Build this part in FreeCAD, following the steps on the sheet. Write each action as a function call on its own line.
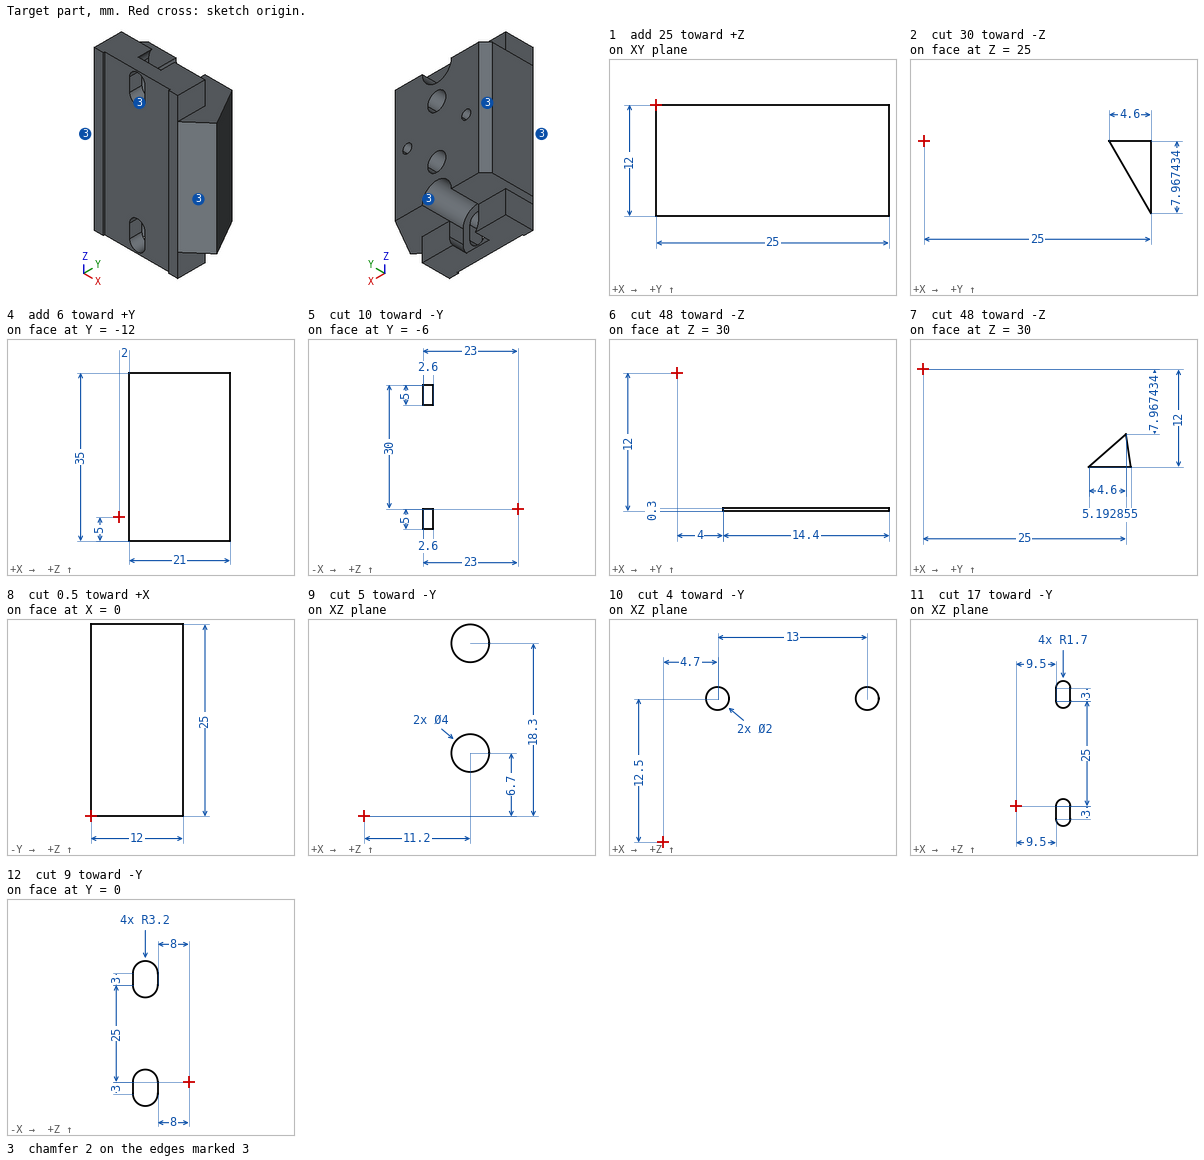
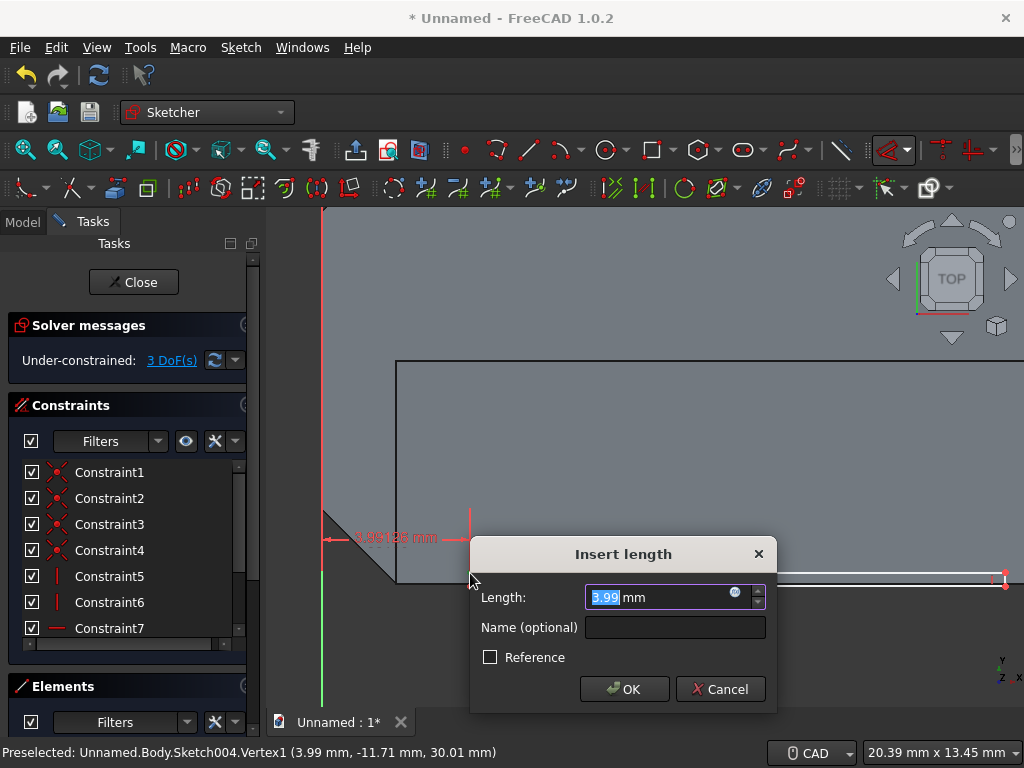
text(4)
key(Return)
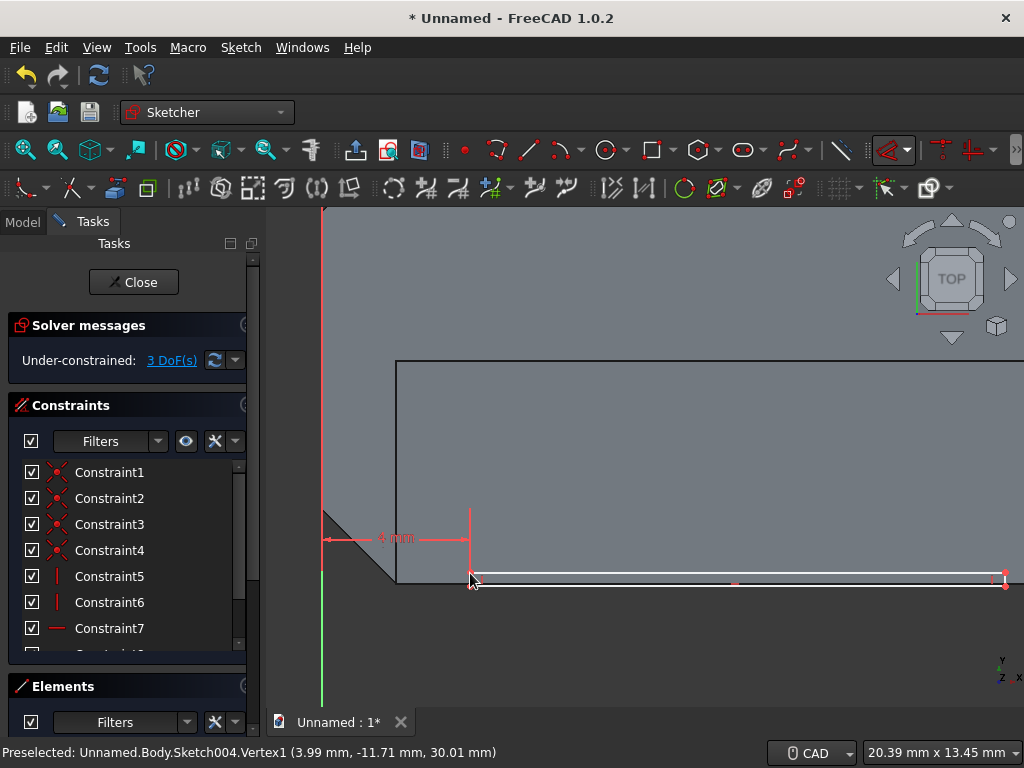
scroll(470, 580, up, 7)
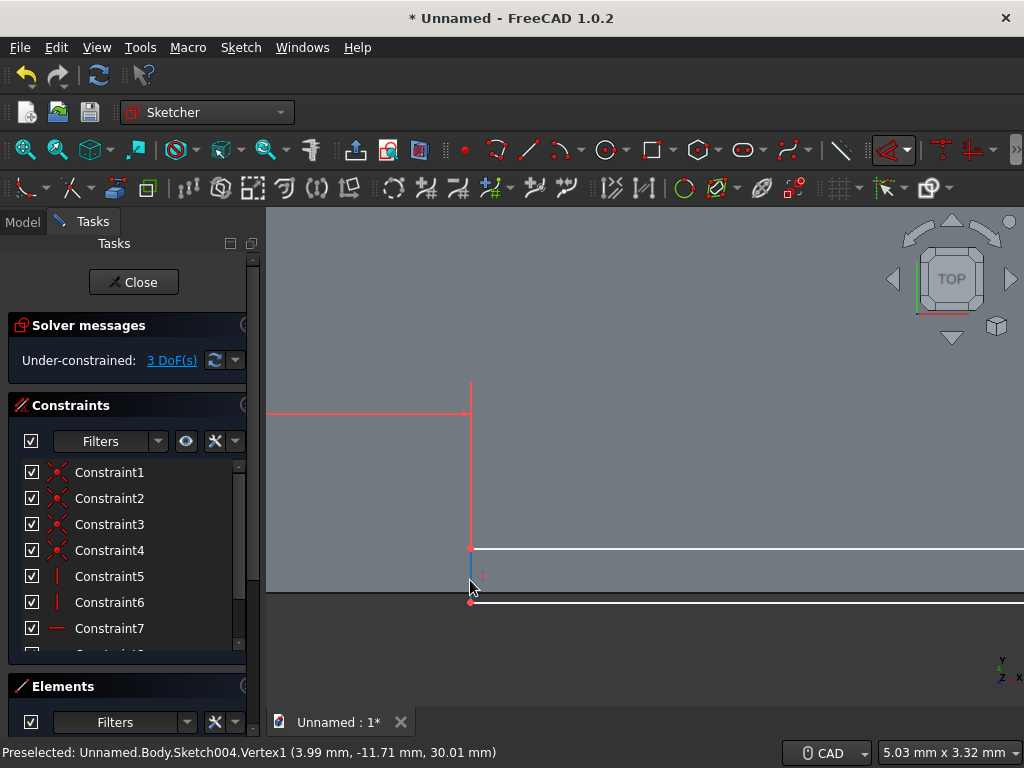
click(471, 576)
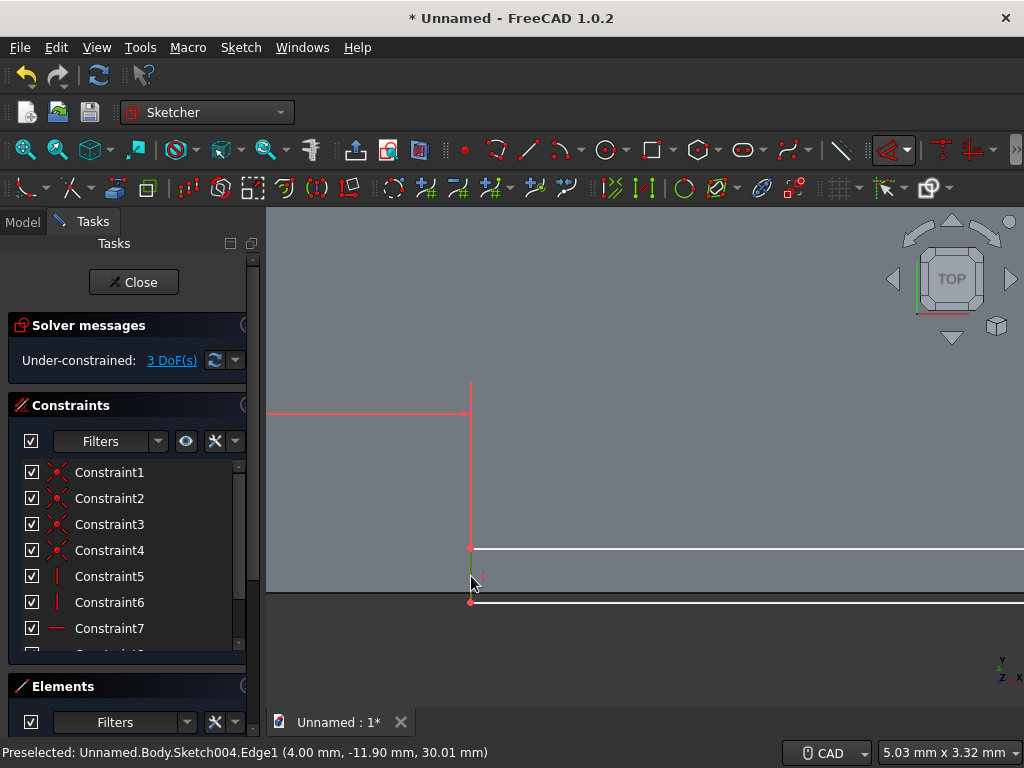
key(i)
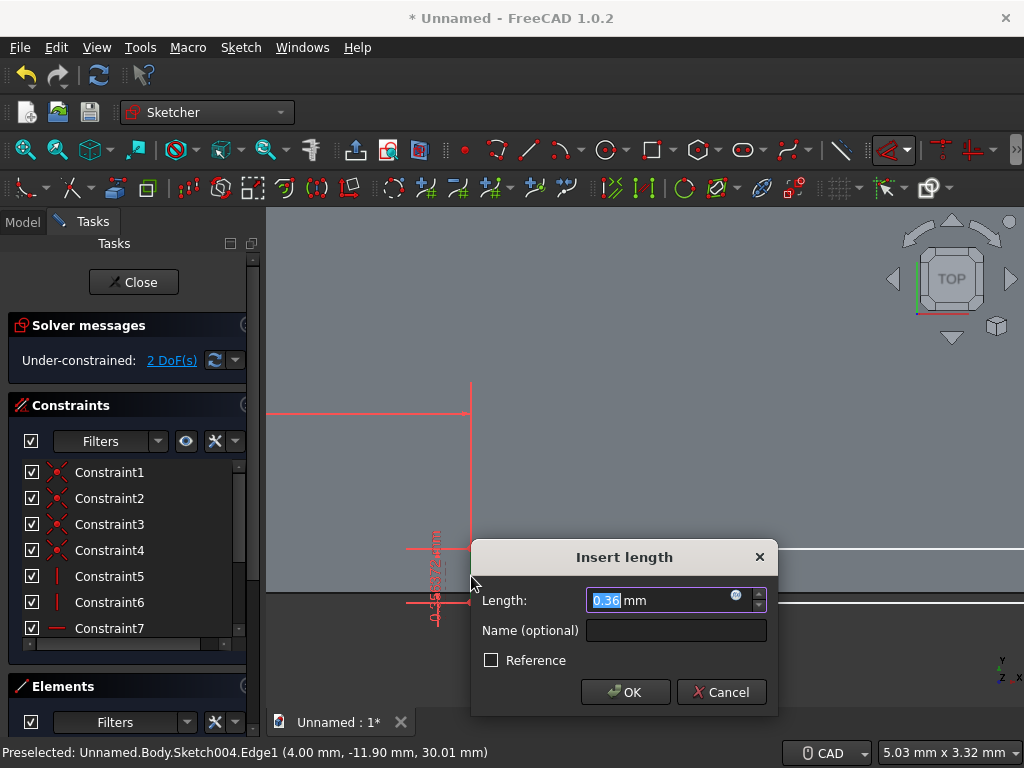
text(0.3)
key(Return)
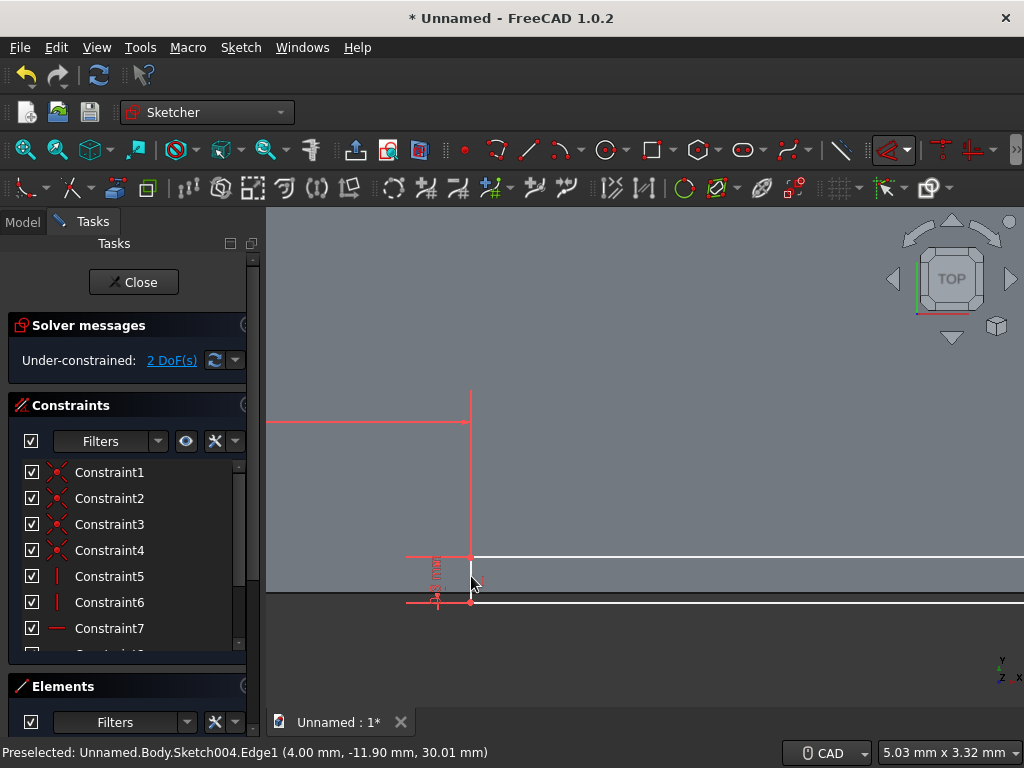
scroll(470, 577, down, 10)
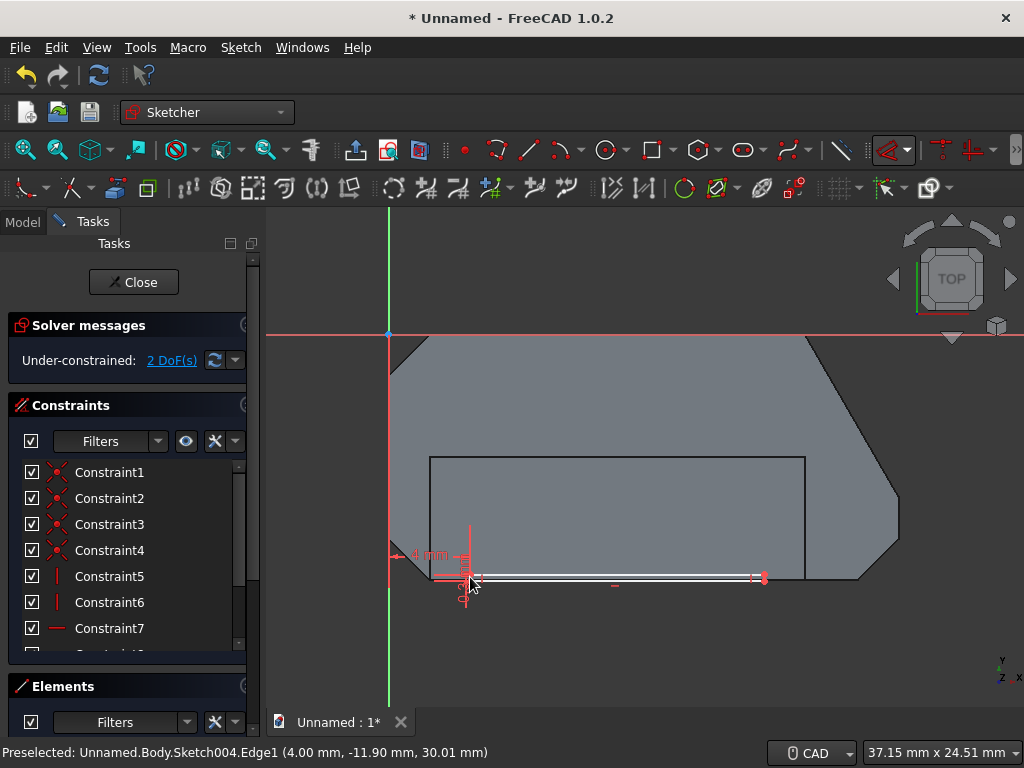
scroll(470, 581, up, 4)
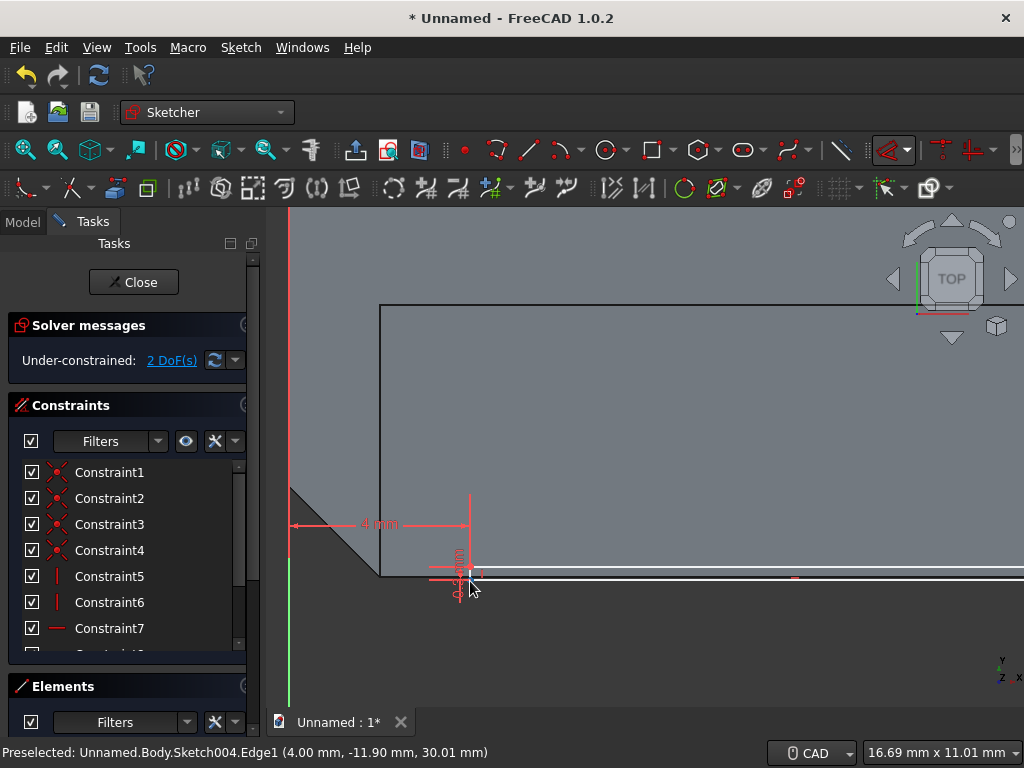
click(470, 580)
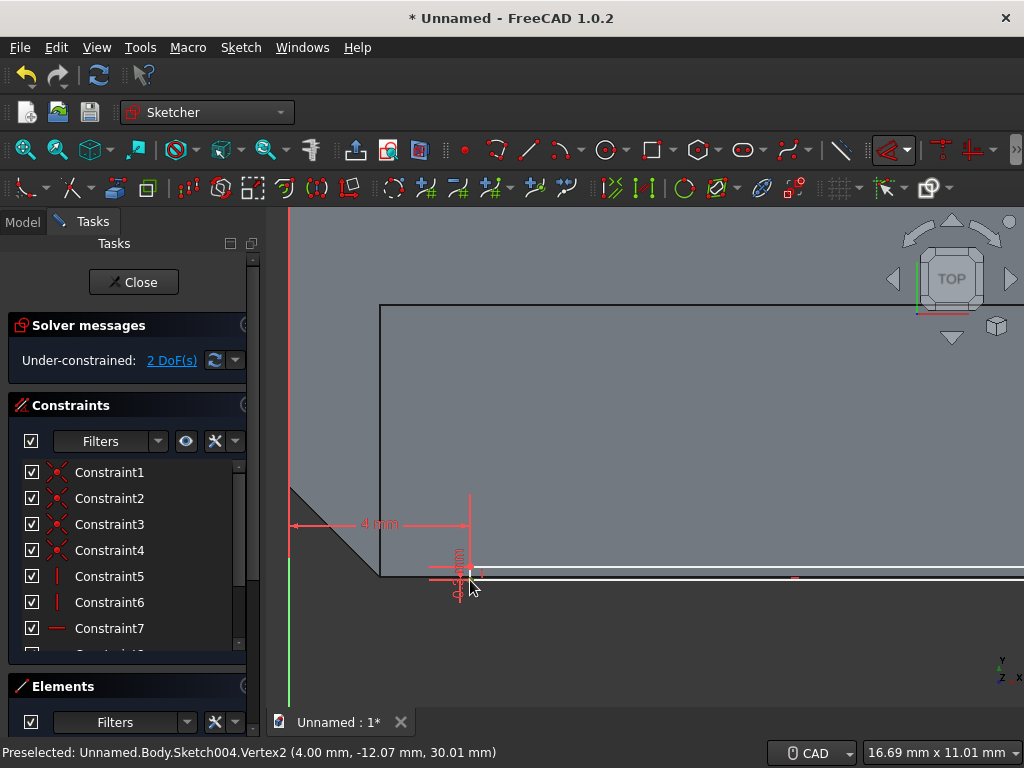
key(i)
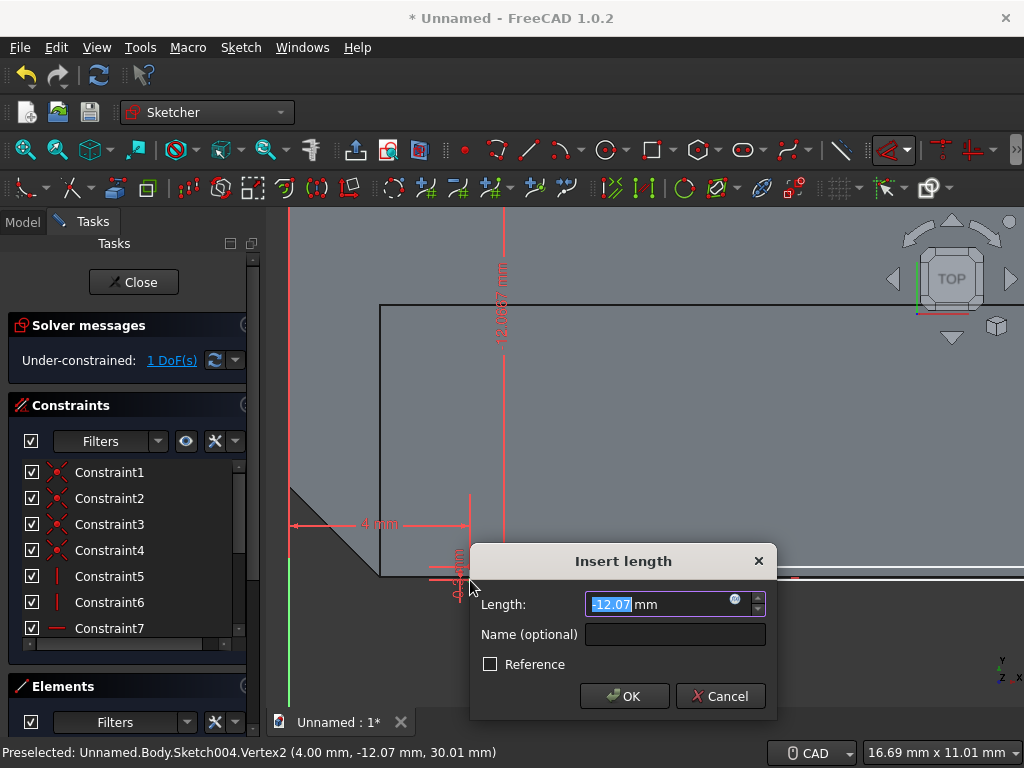
text(-12)
key(Return)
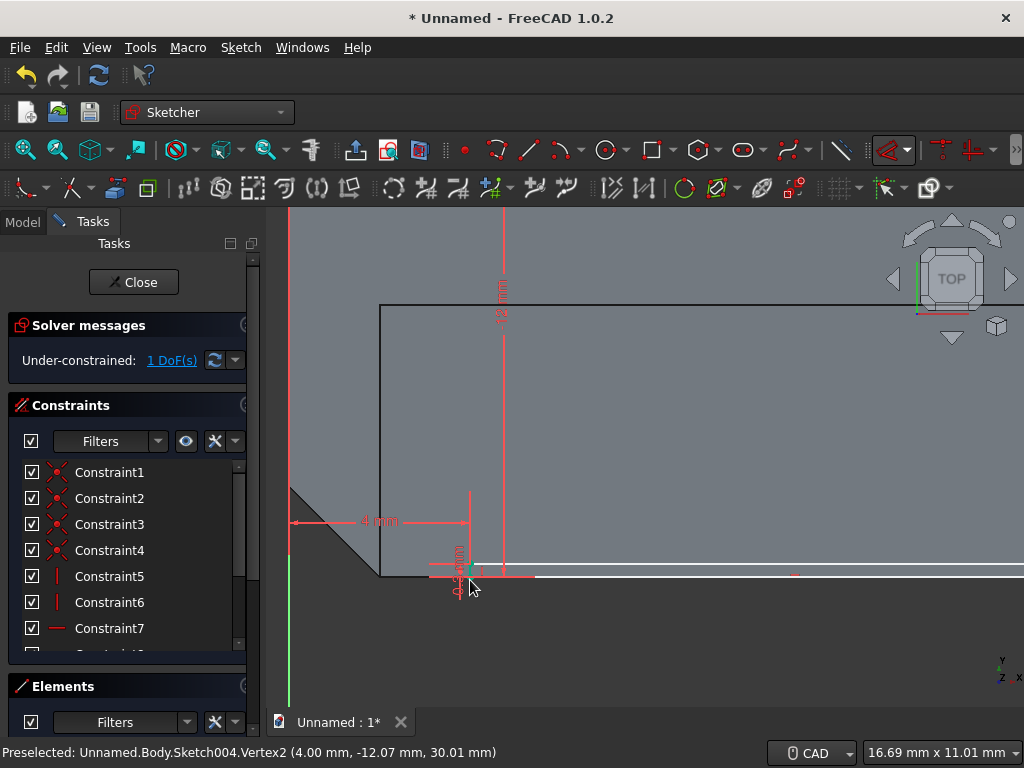
click(667, 577)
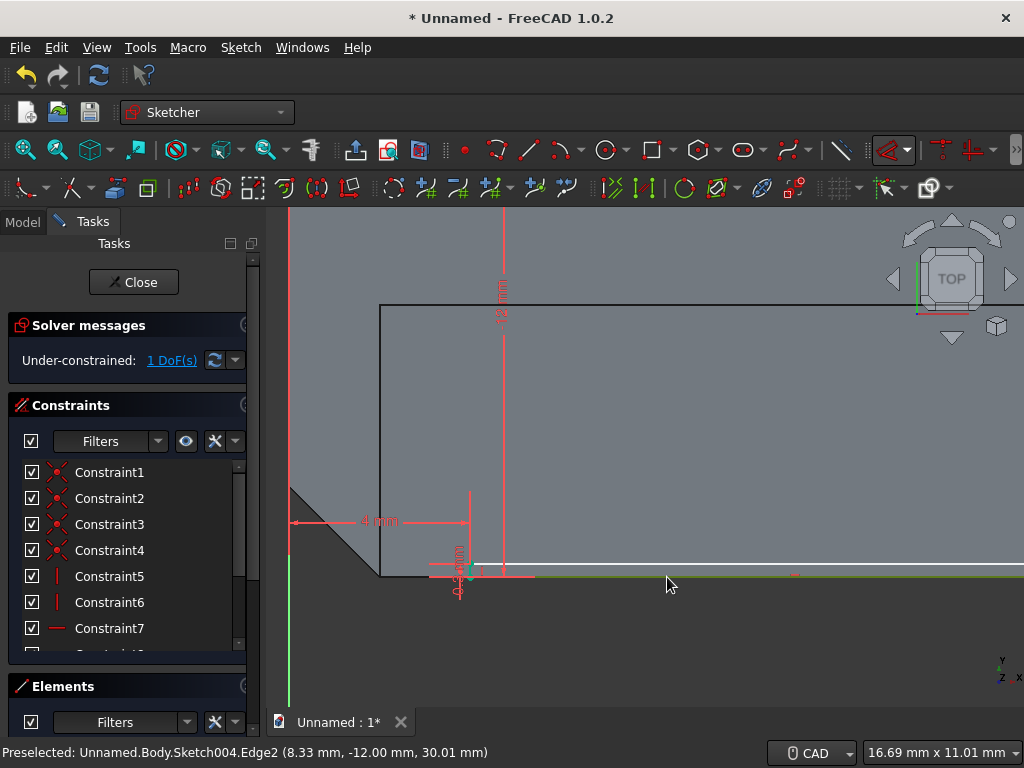
click(910, 150)